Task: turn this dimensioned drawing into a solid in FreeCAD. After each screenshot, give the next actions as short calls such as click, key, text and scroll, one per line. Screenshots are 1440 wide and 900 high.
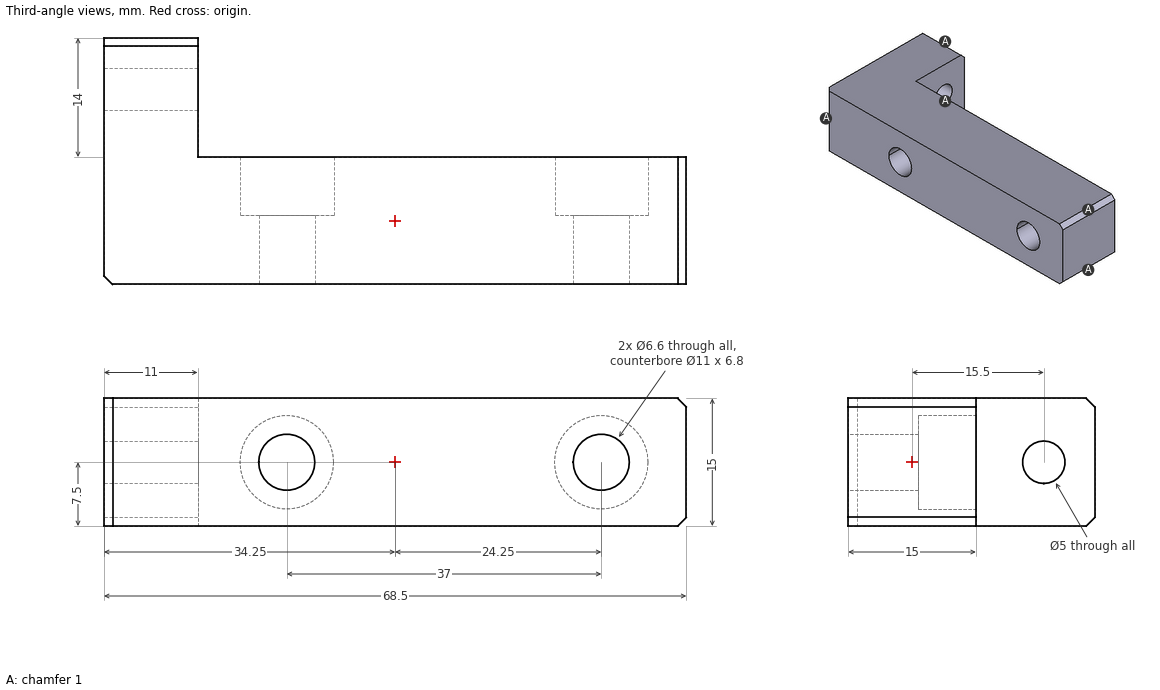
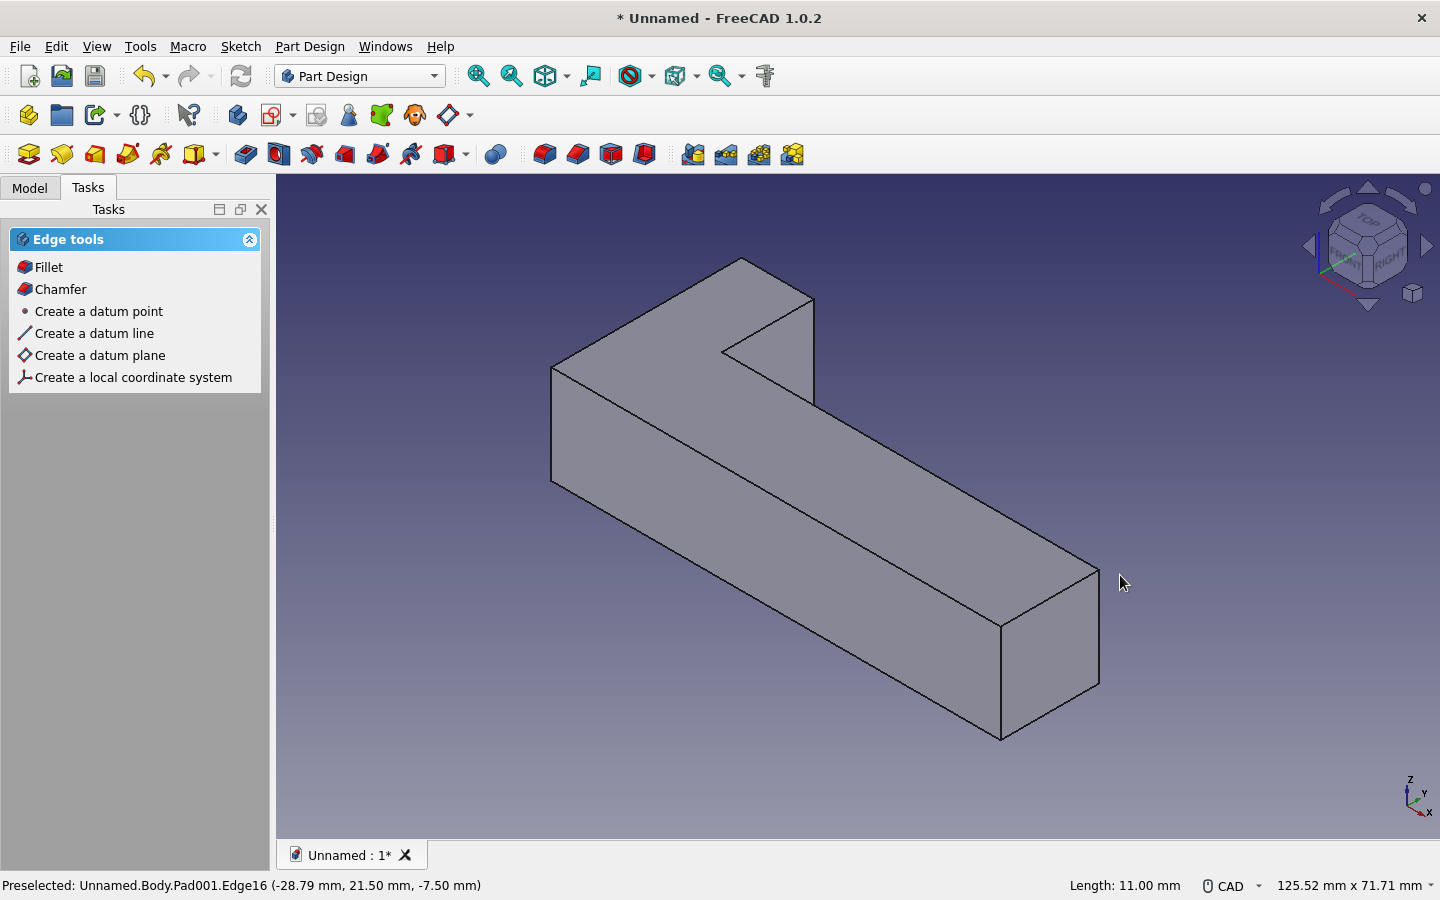
click(1050, 597, ctrl)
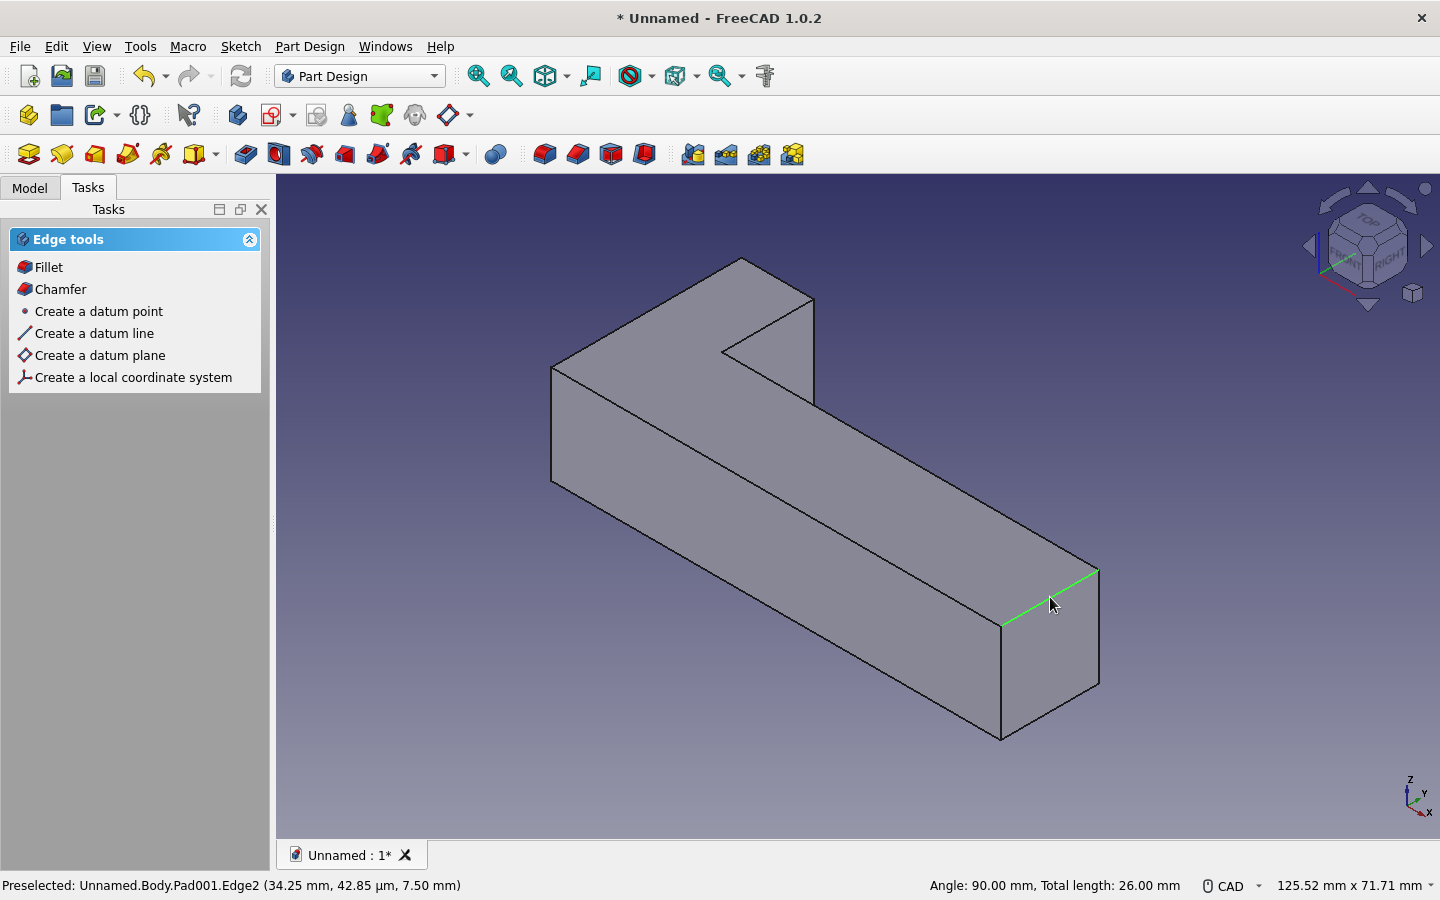
key(2)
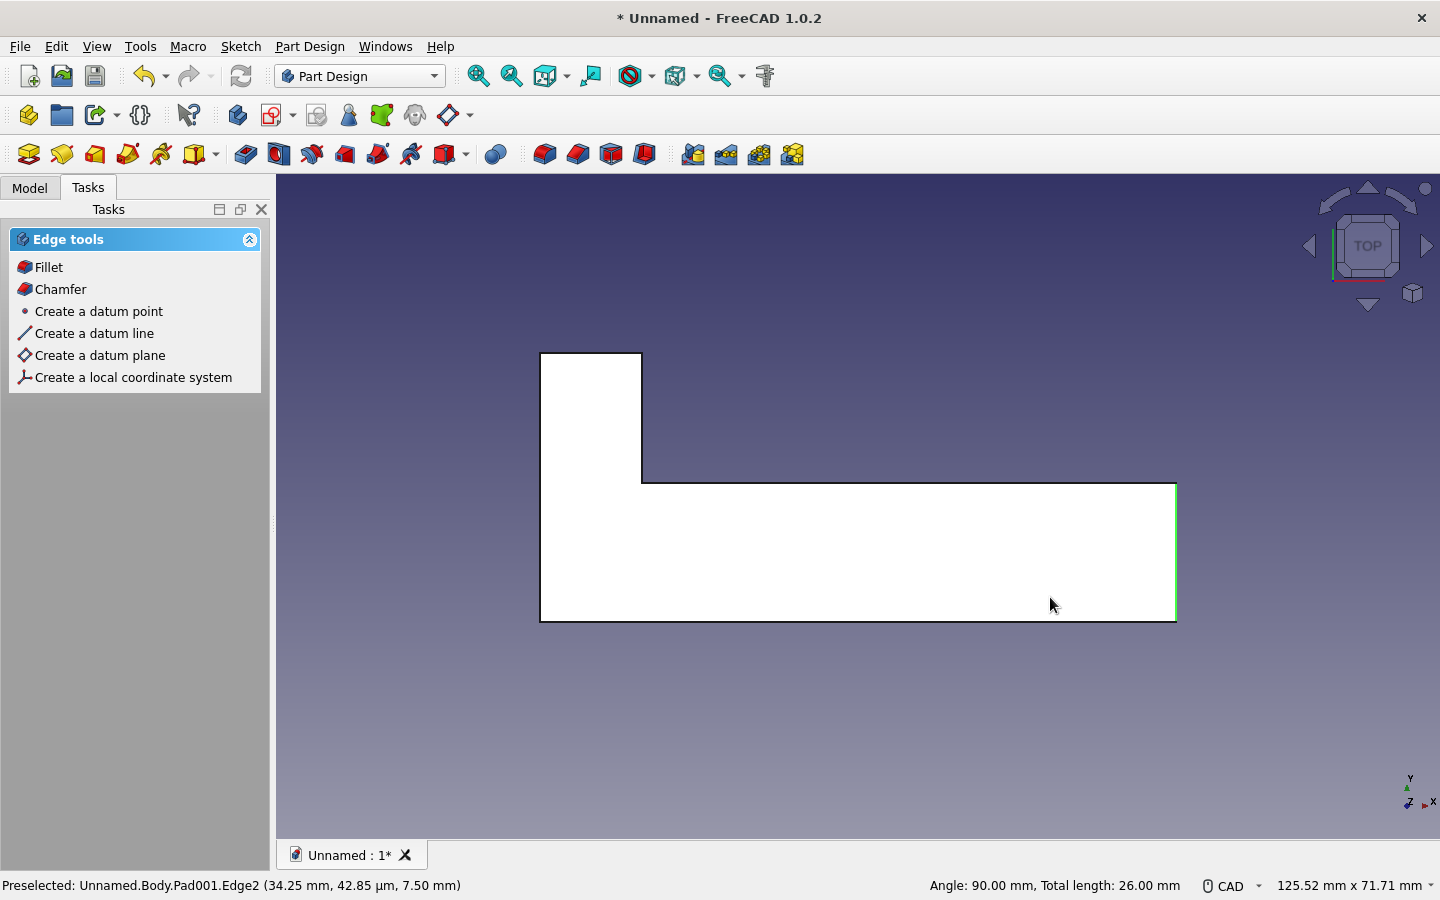
click(591, 352, ctrl)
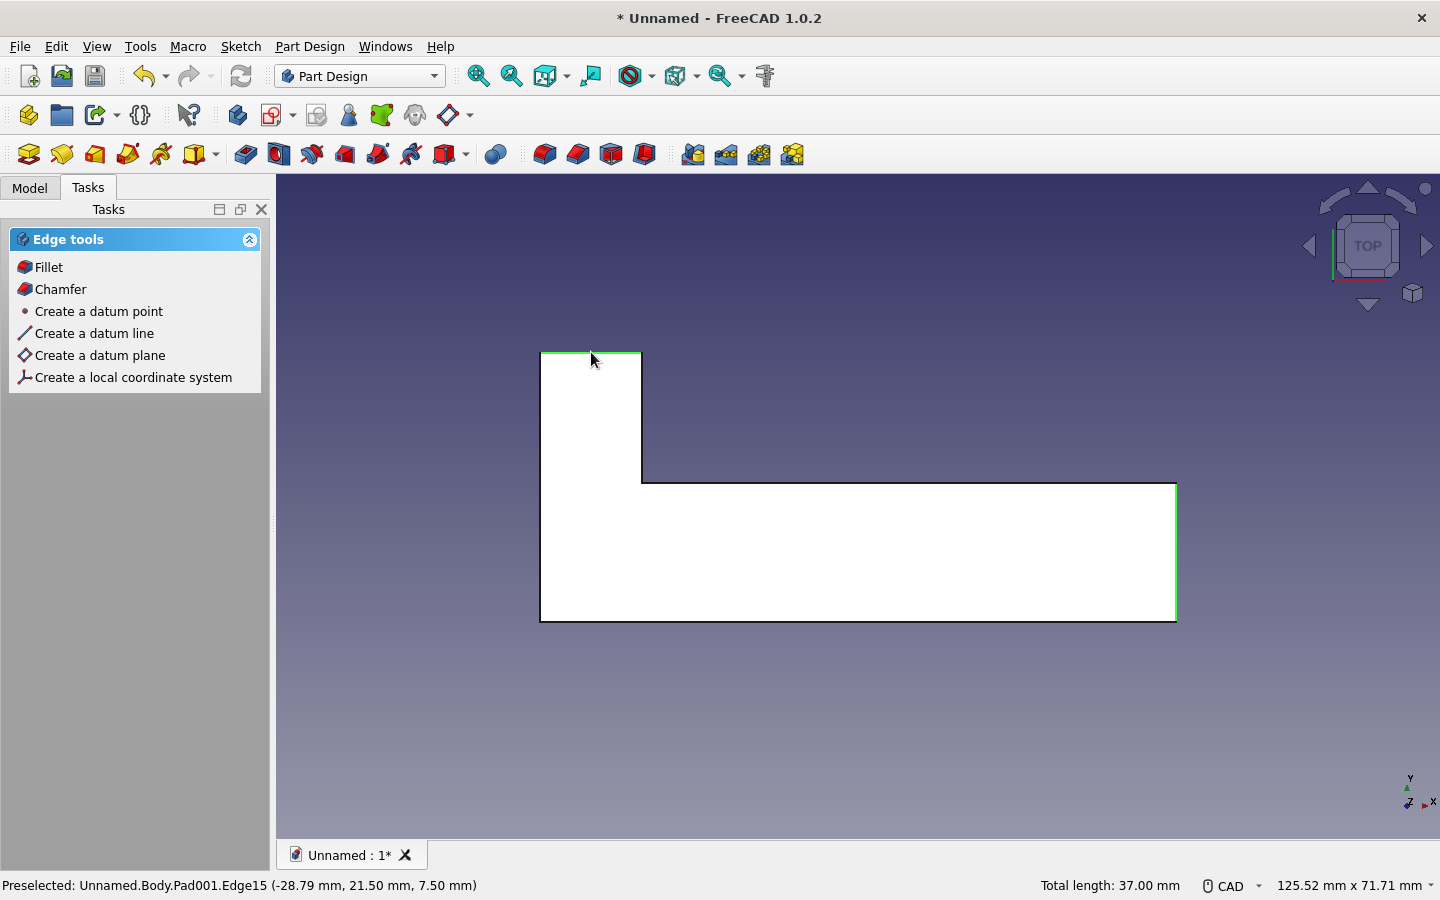
key(1)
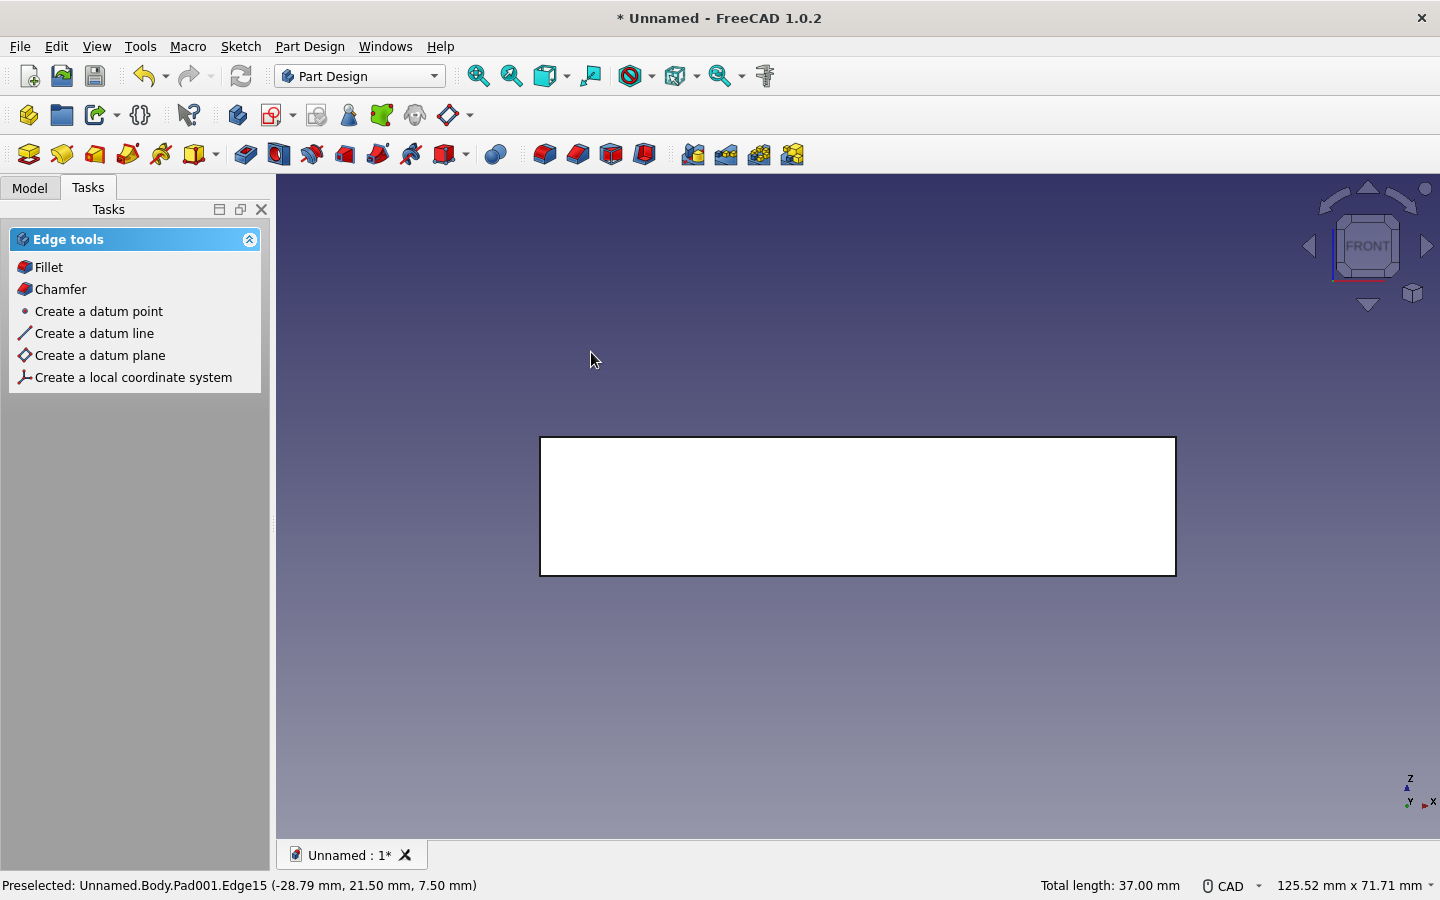
click(540, 506, ctrl)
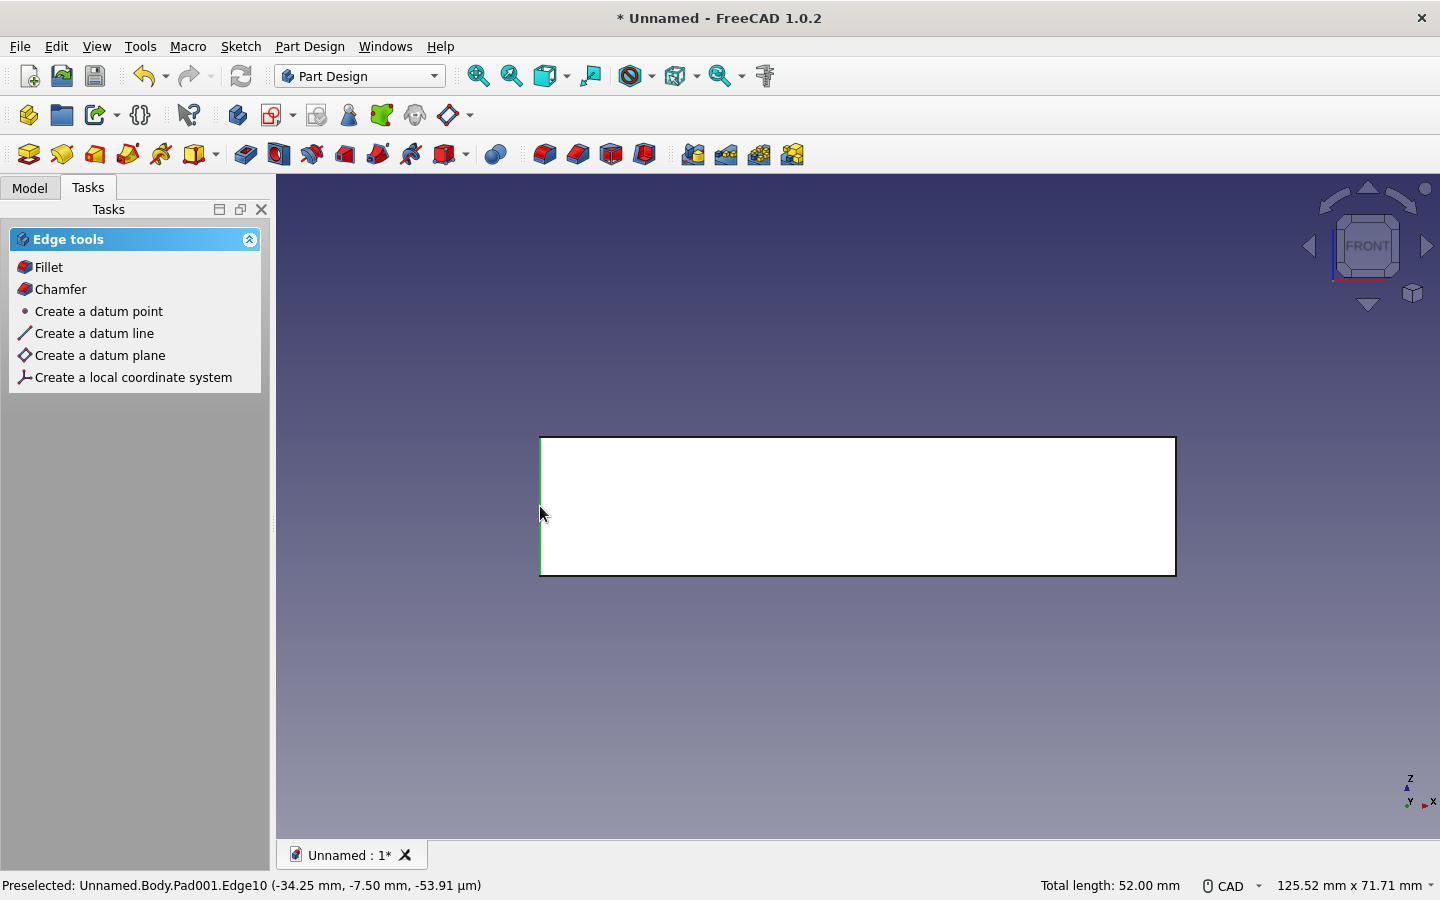
key(3)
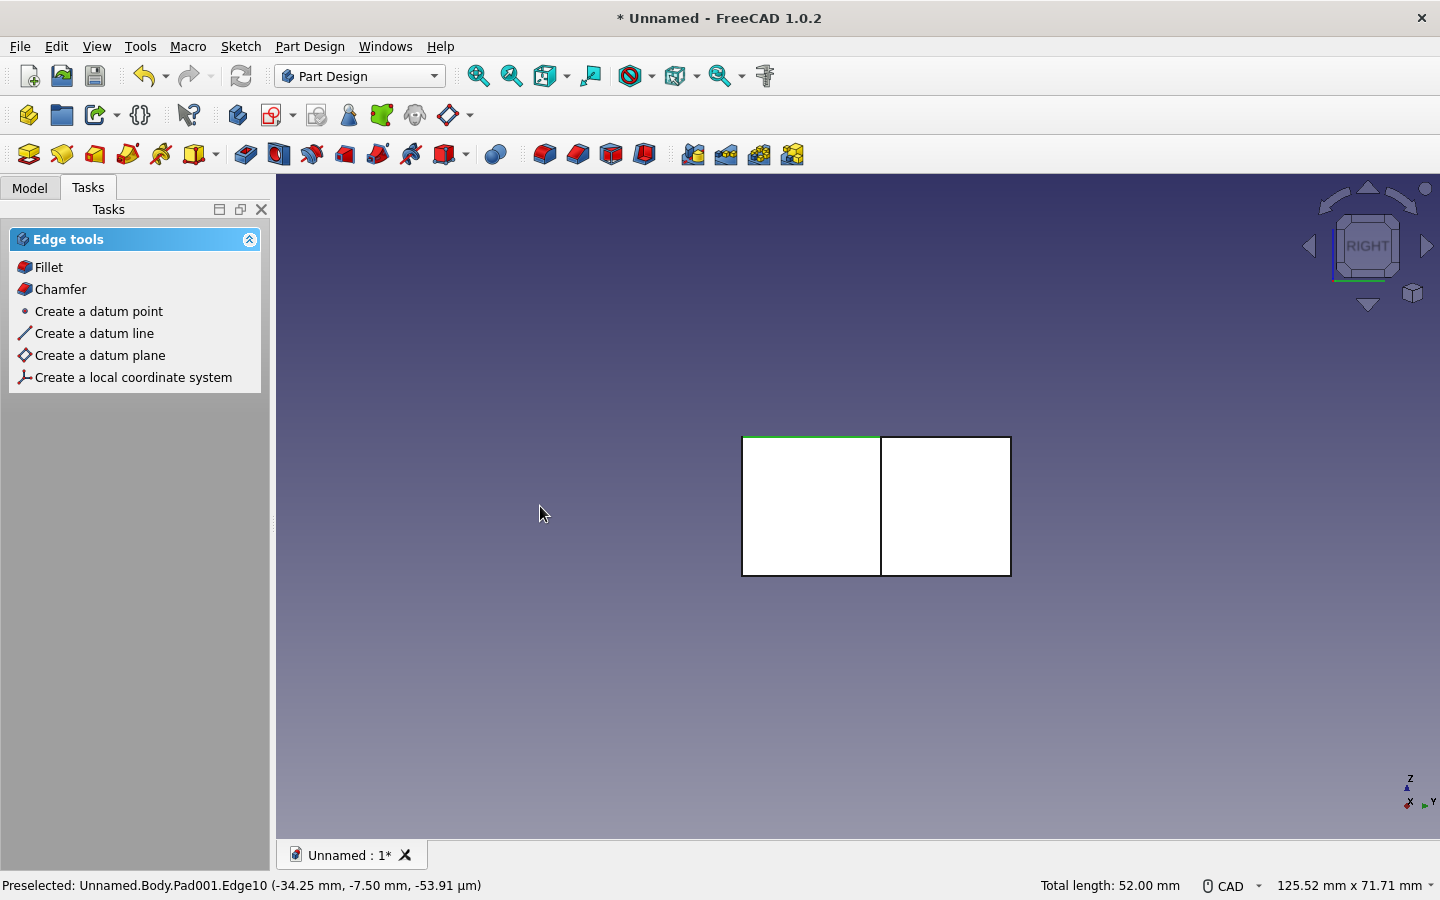
click(479, 76)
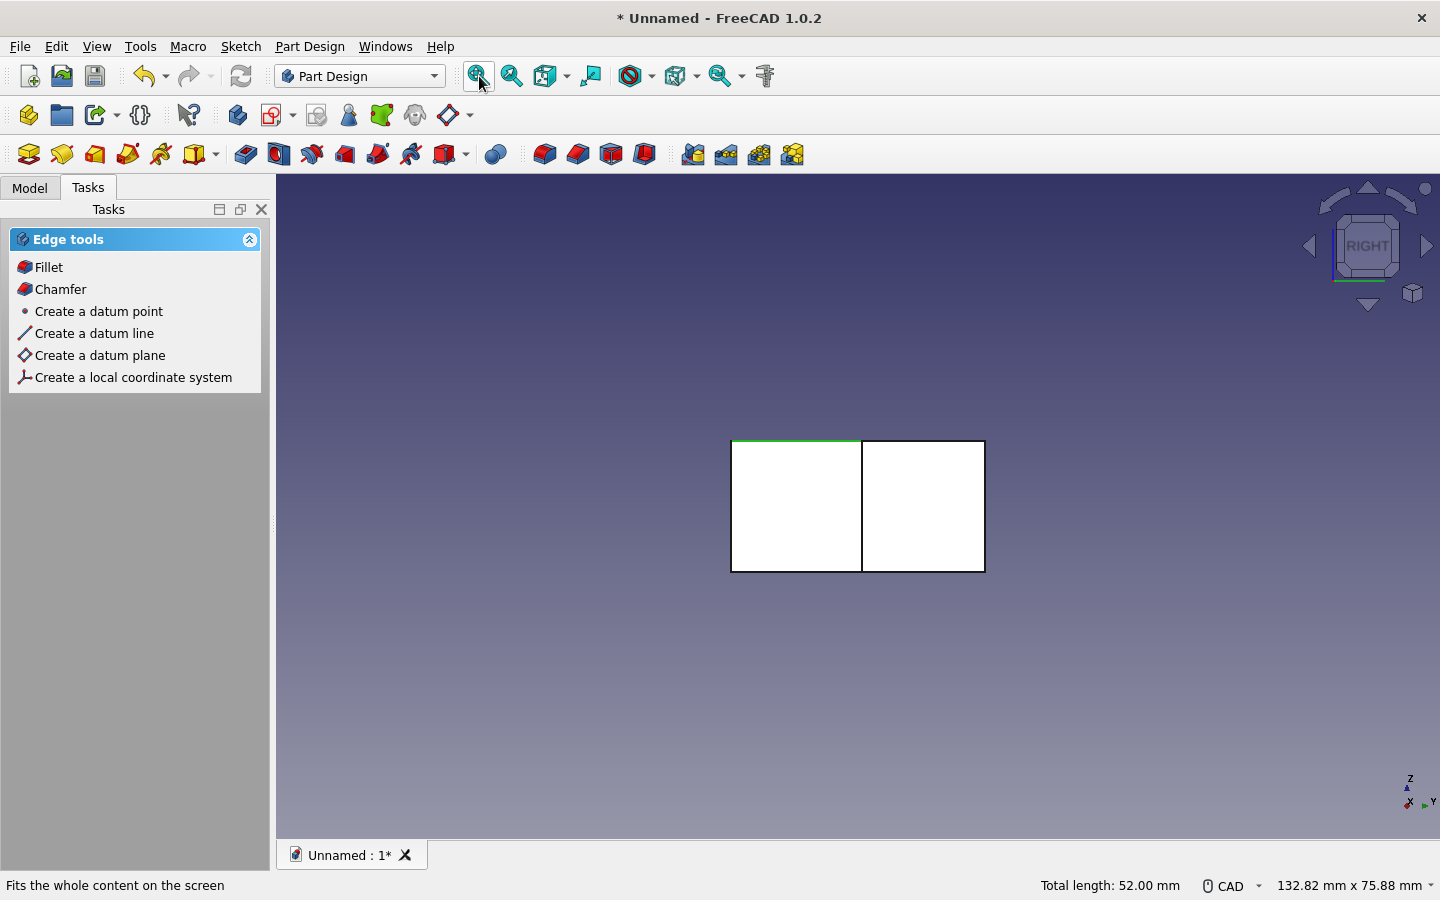
click(797, 571, ctrl)